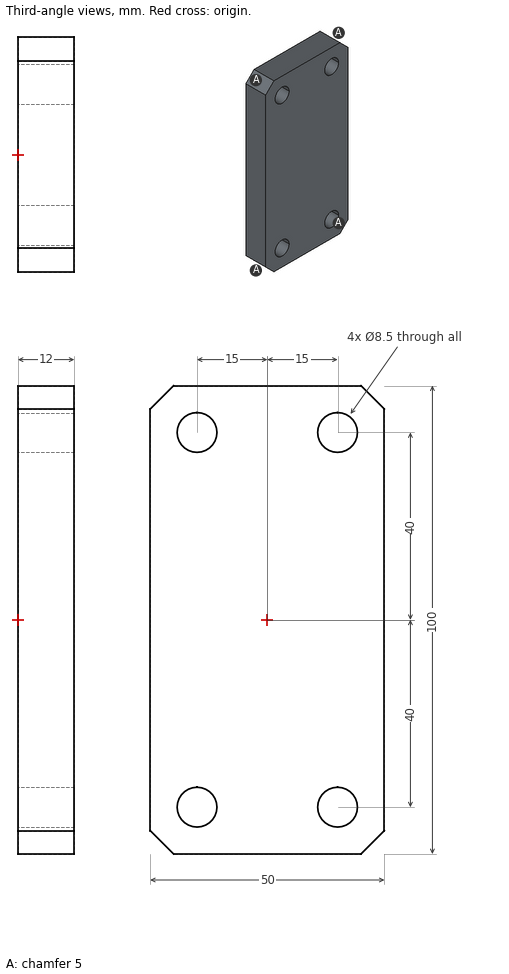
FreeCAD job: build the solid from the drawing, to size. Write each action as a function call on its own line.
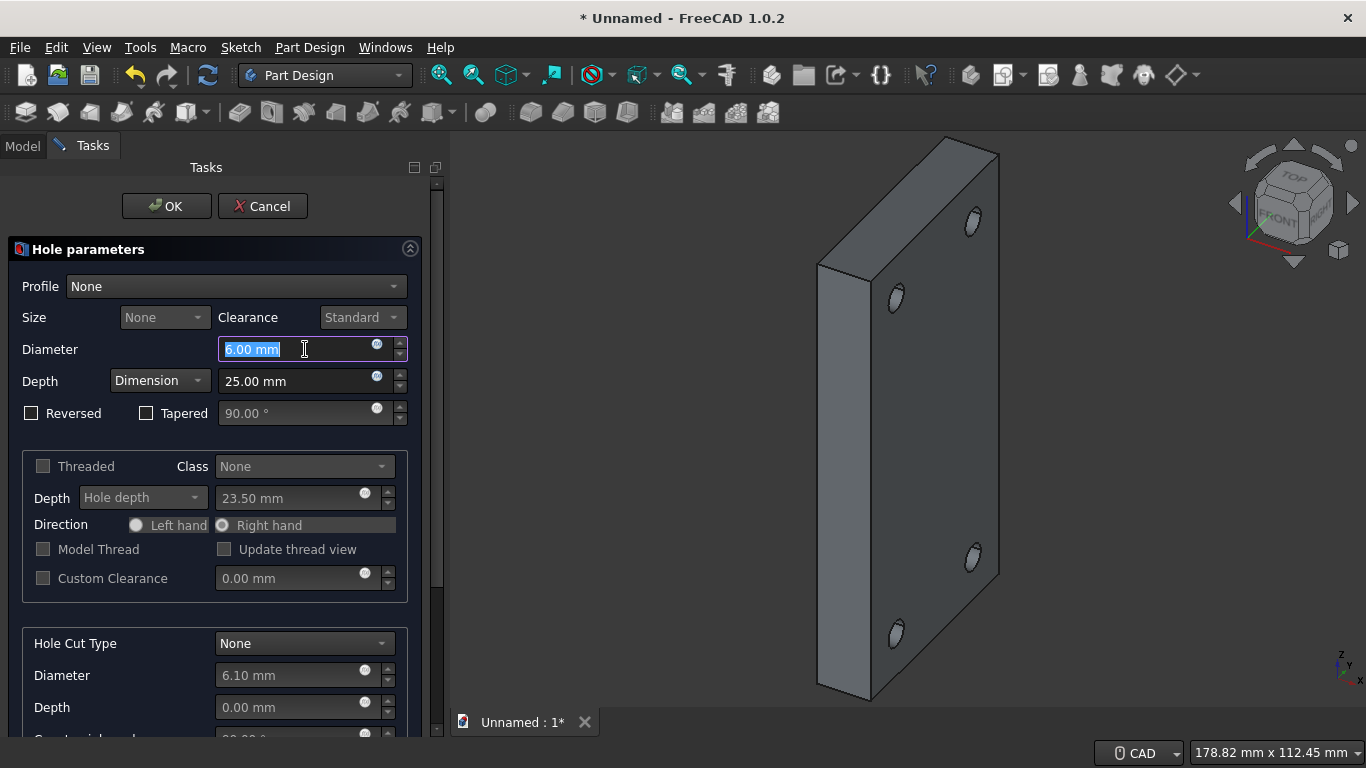
text(8.5)
key(Tab)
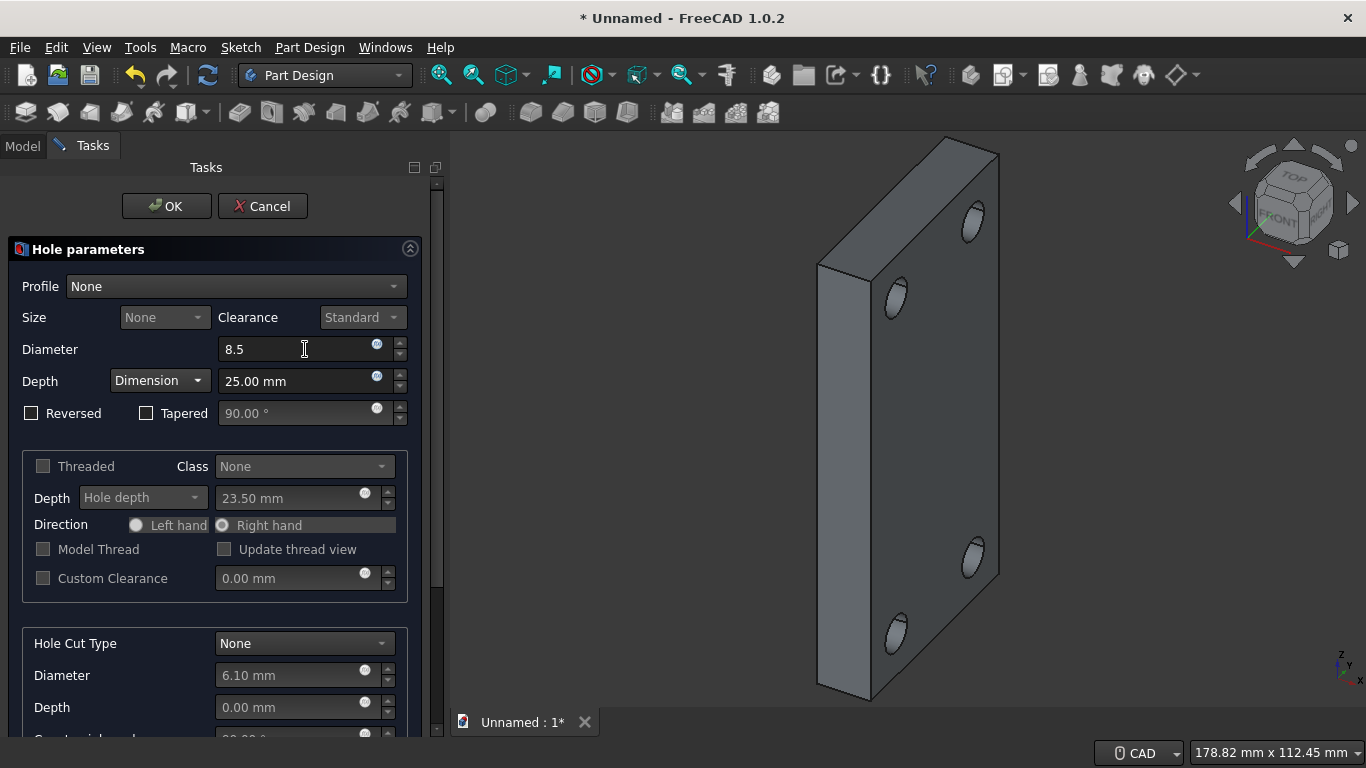
click(161, 380)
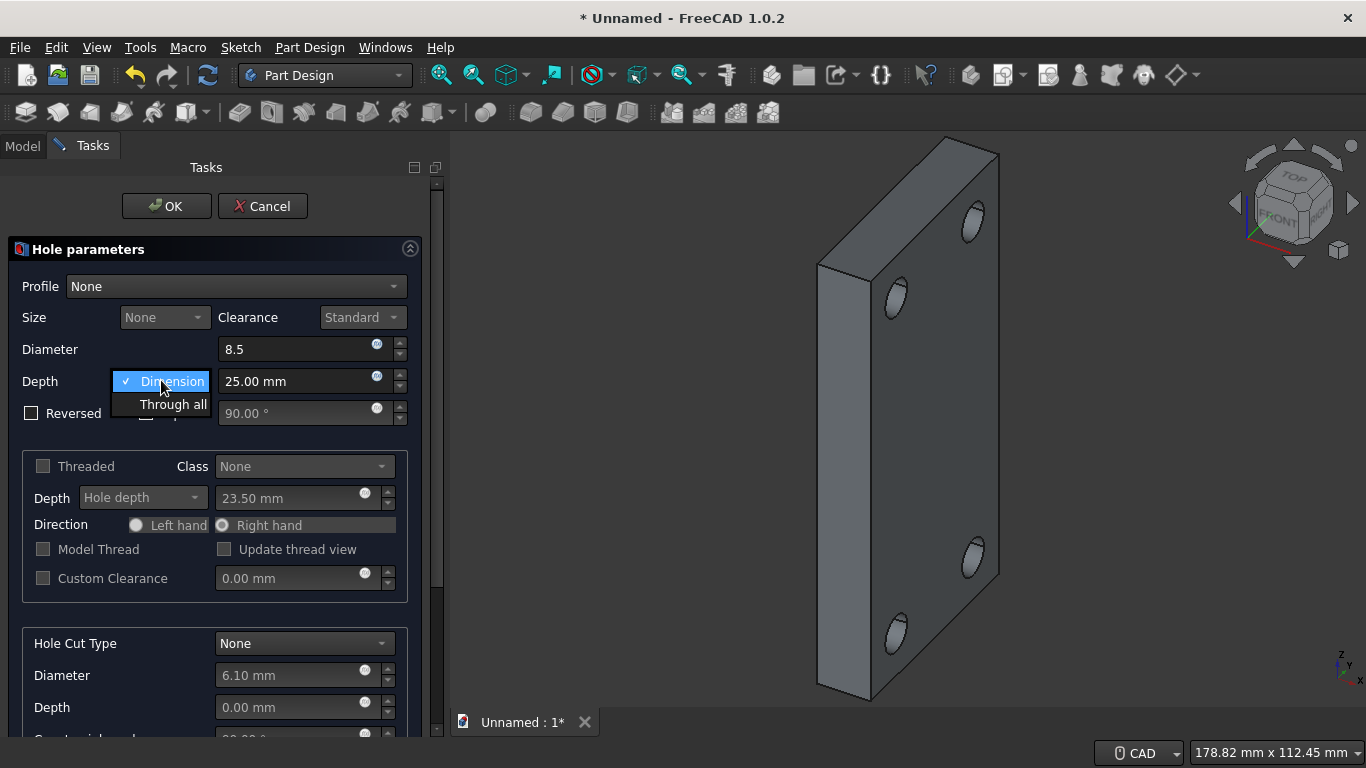
click(160, 404)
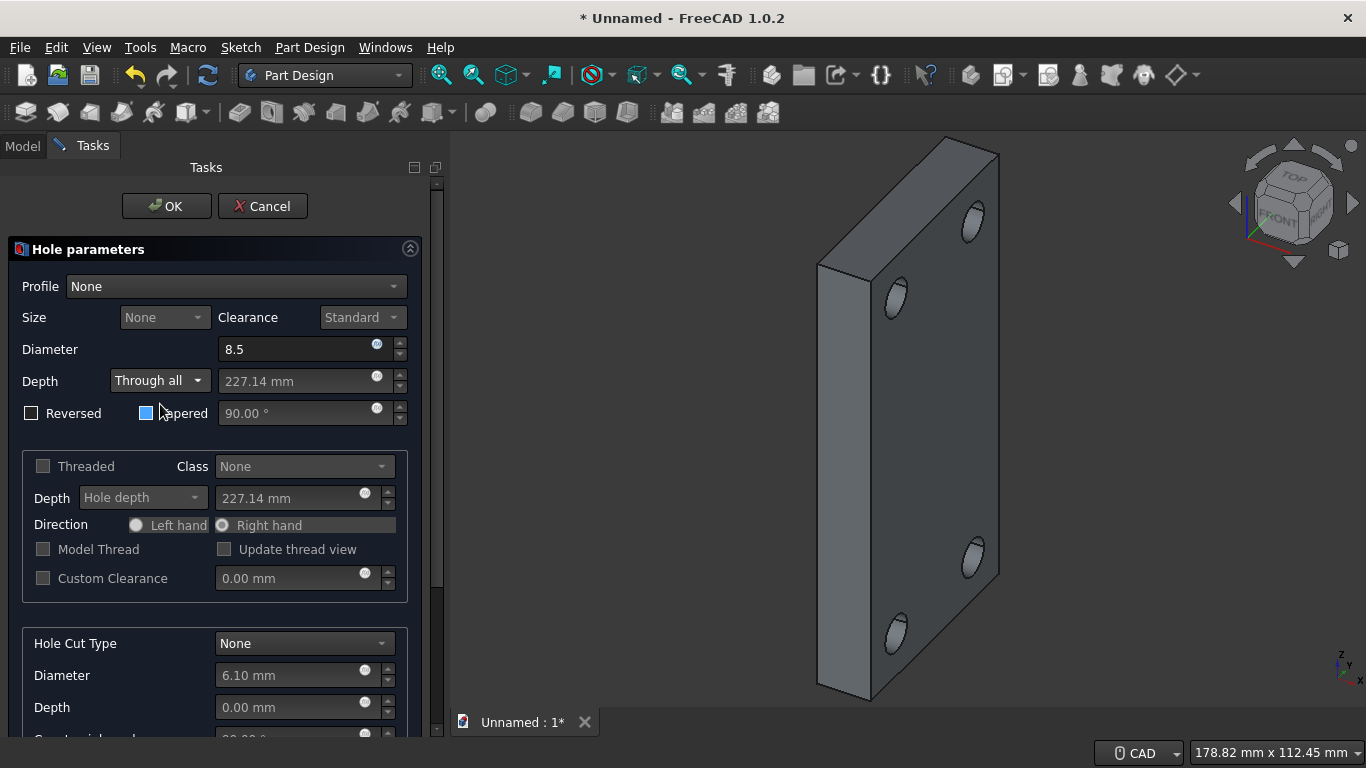
click(167, 206)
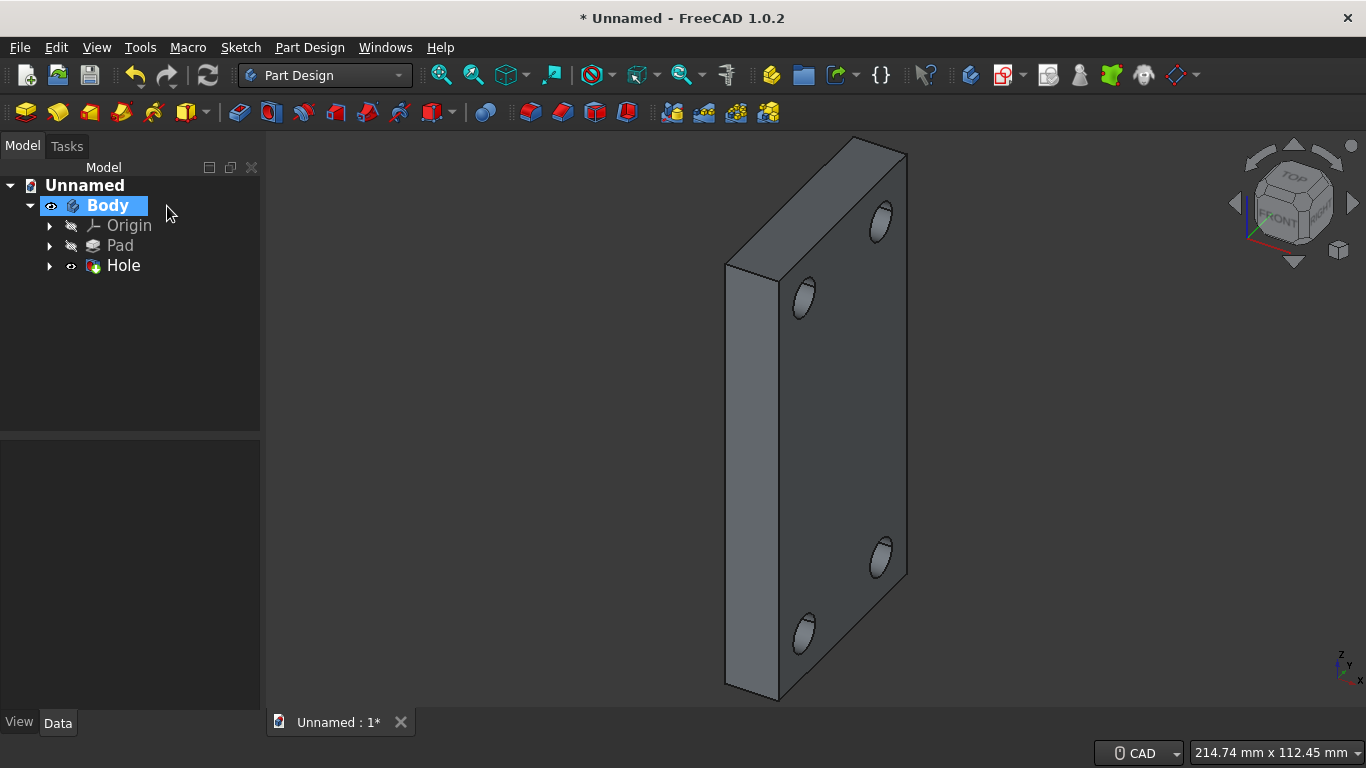
click(752, 272)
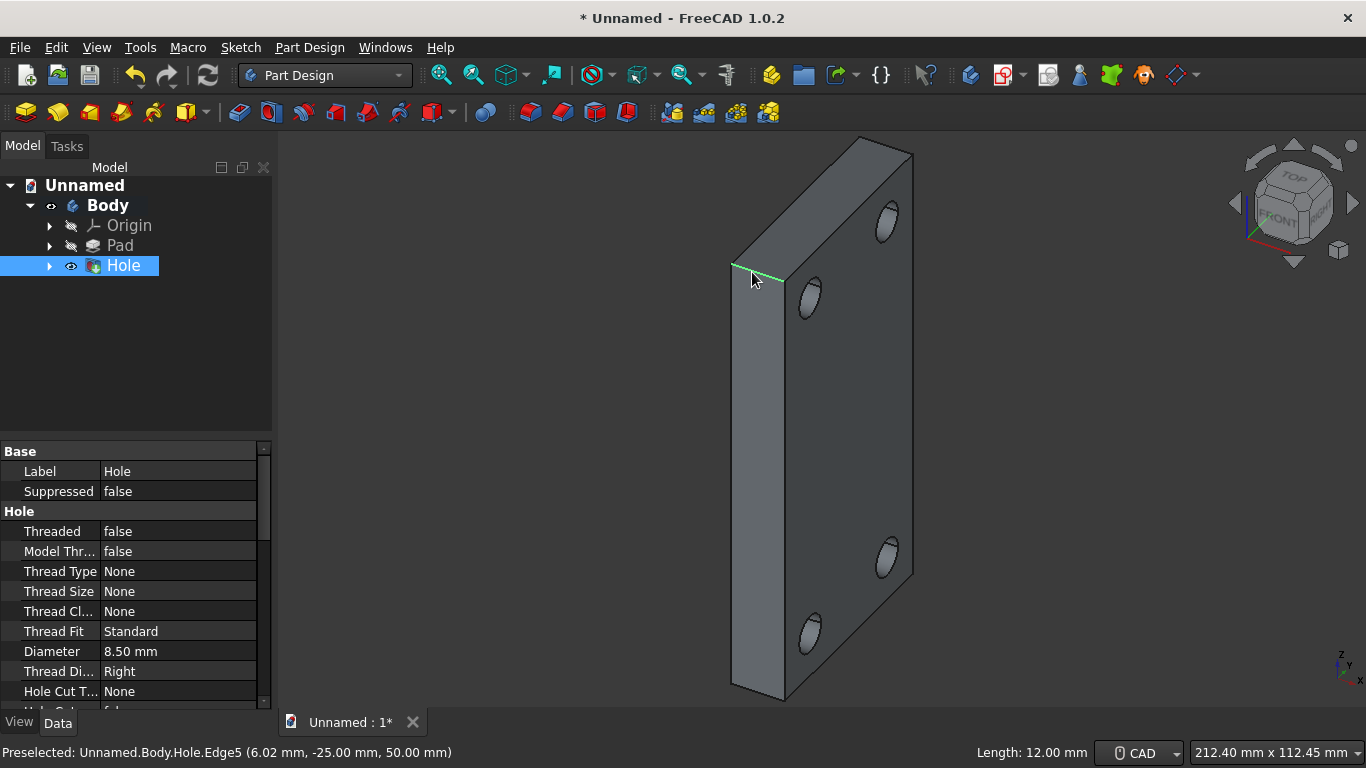
key(0)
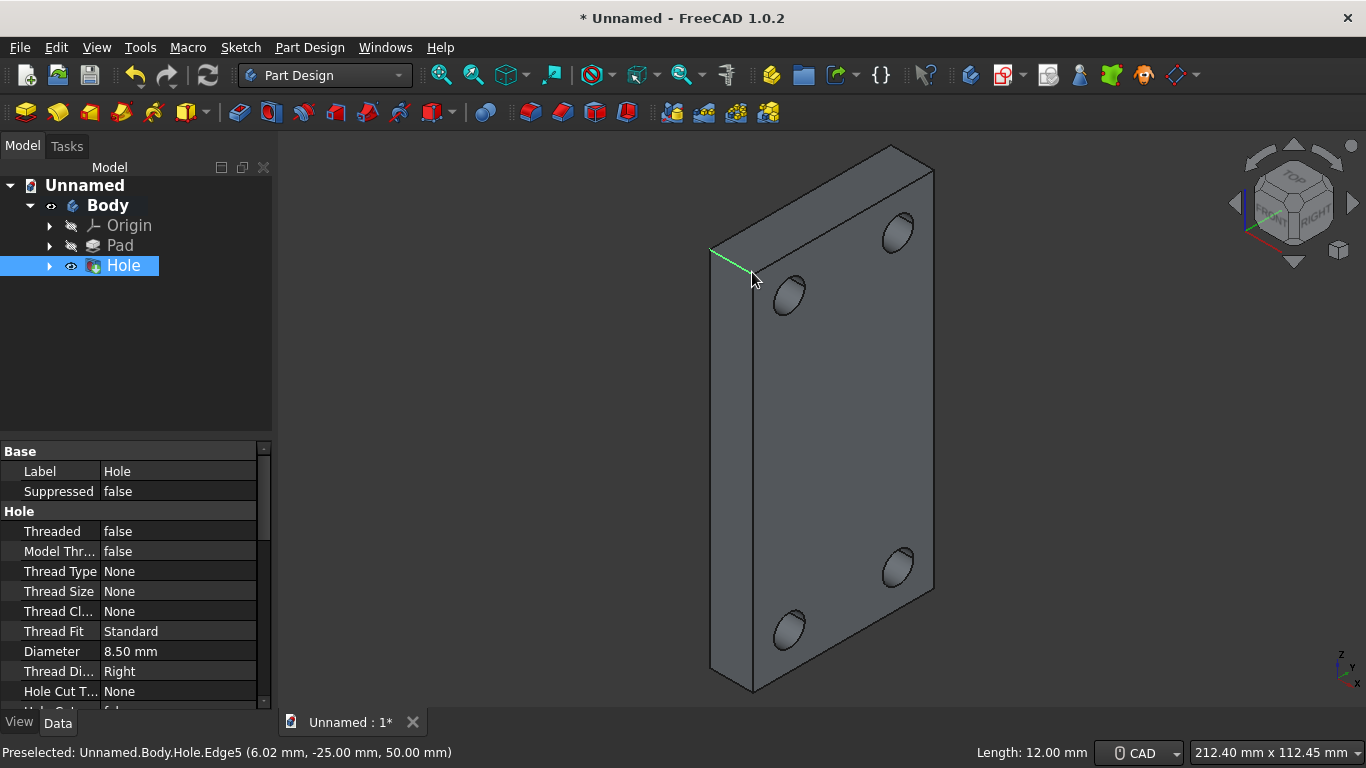
key(2)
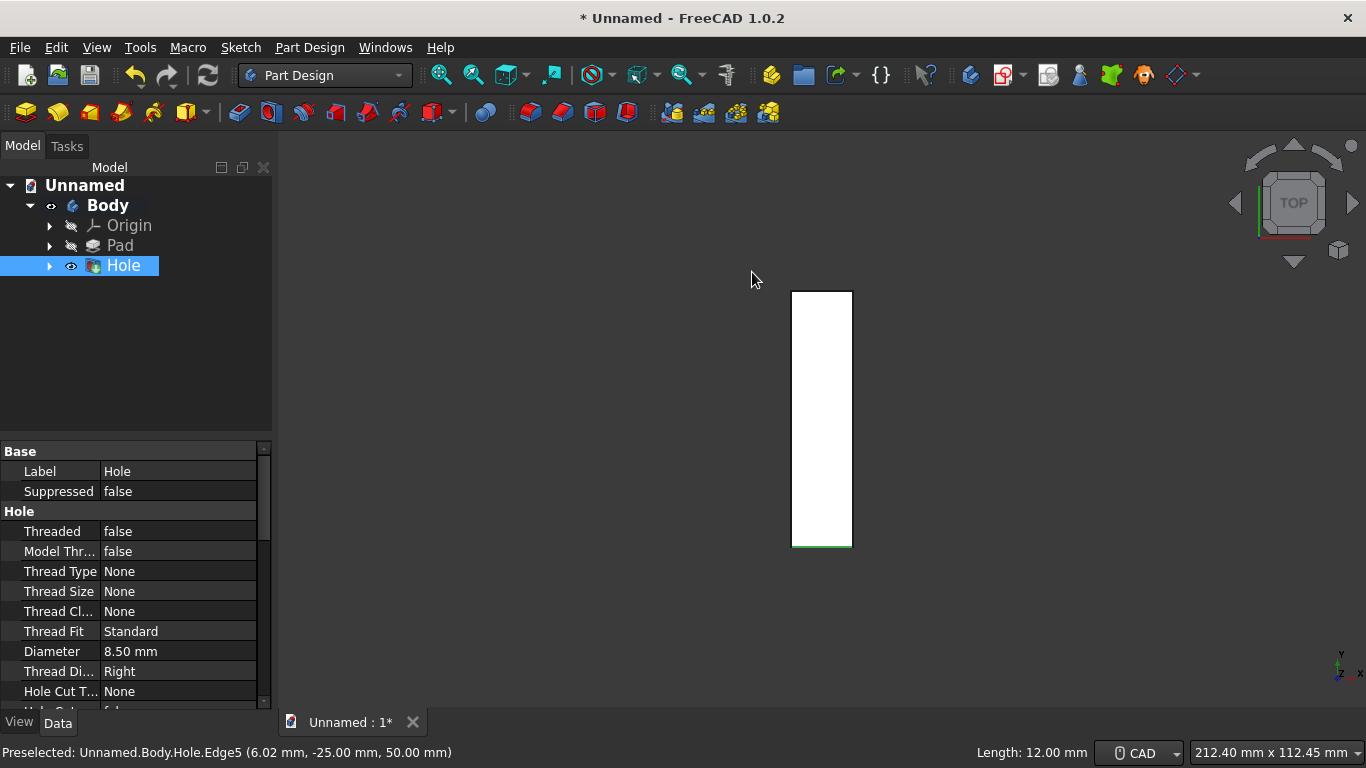
click(442, 76)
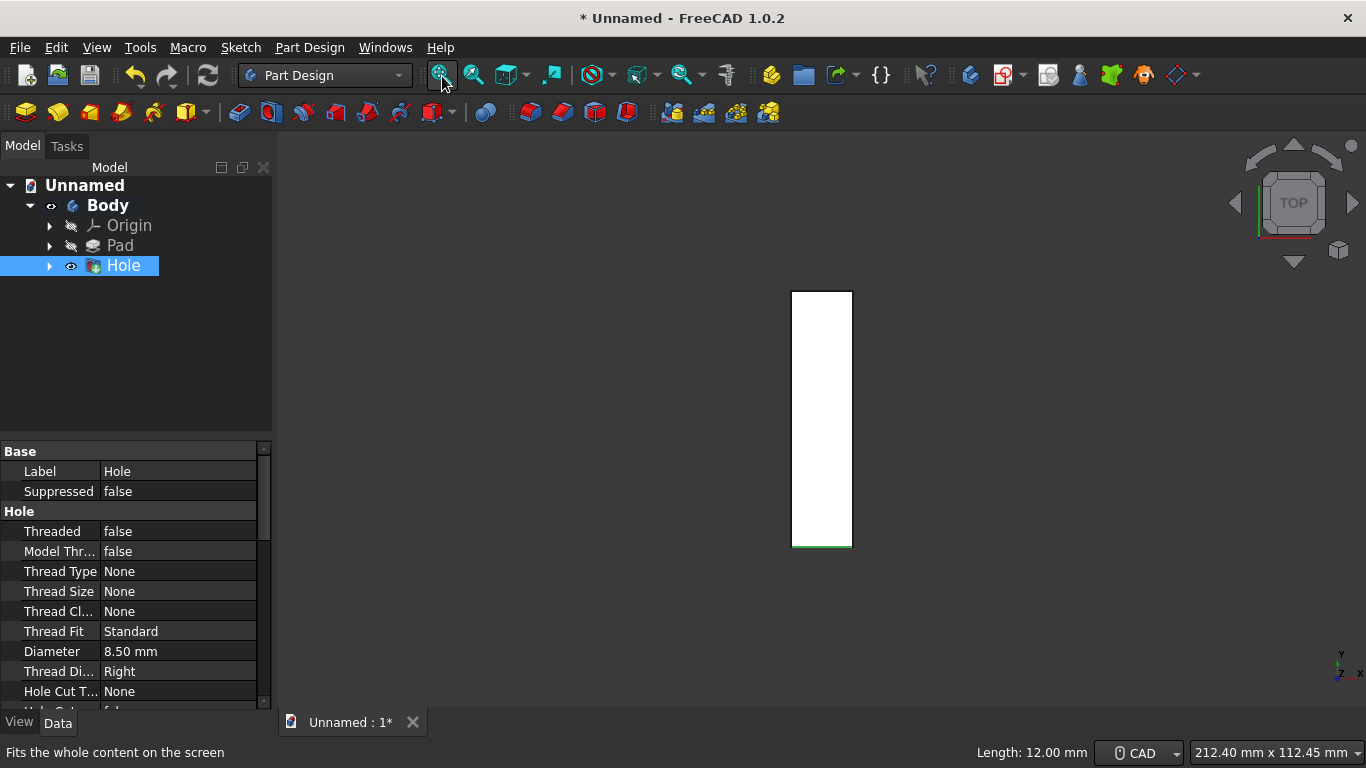
click(822, 290, ctrl)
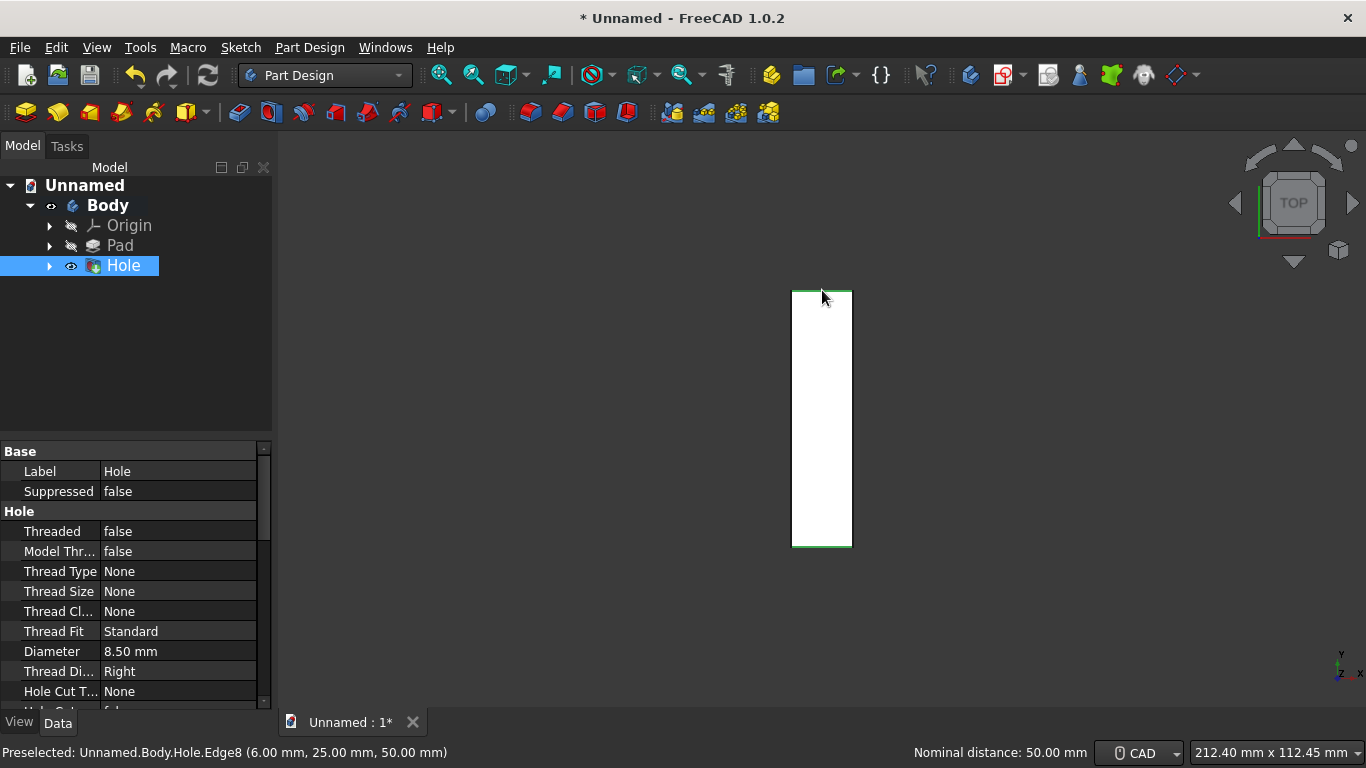
key(1)